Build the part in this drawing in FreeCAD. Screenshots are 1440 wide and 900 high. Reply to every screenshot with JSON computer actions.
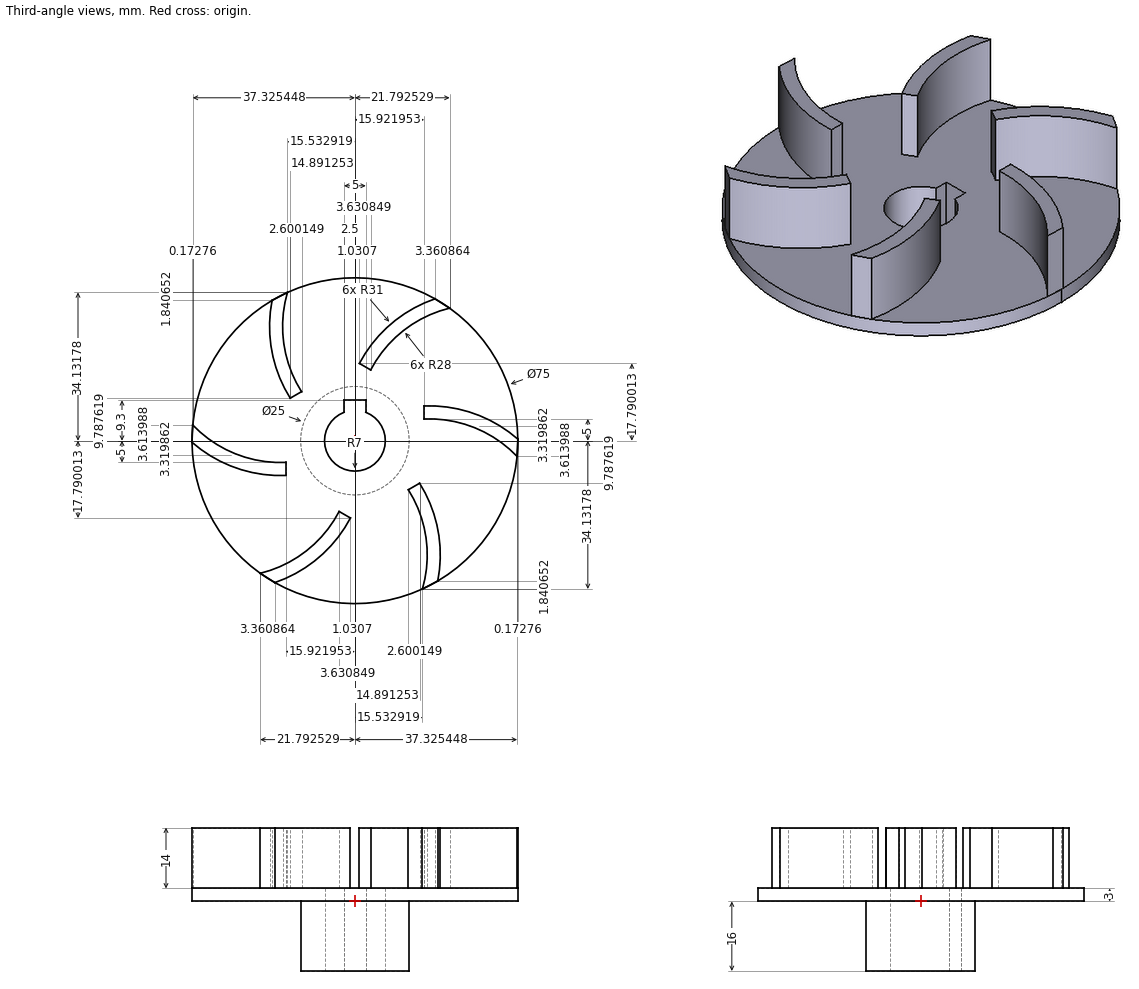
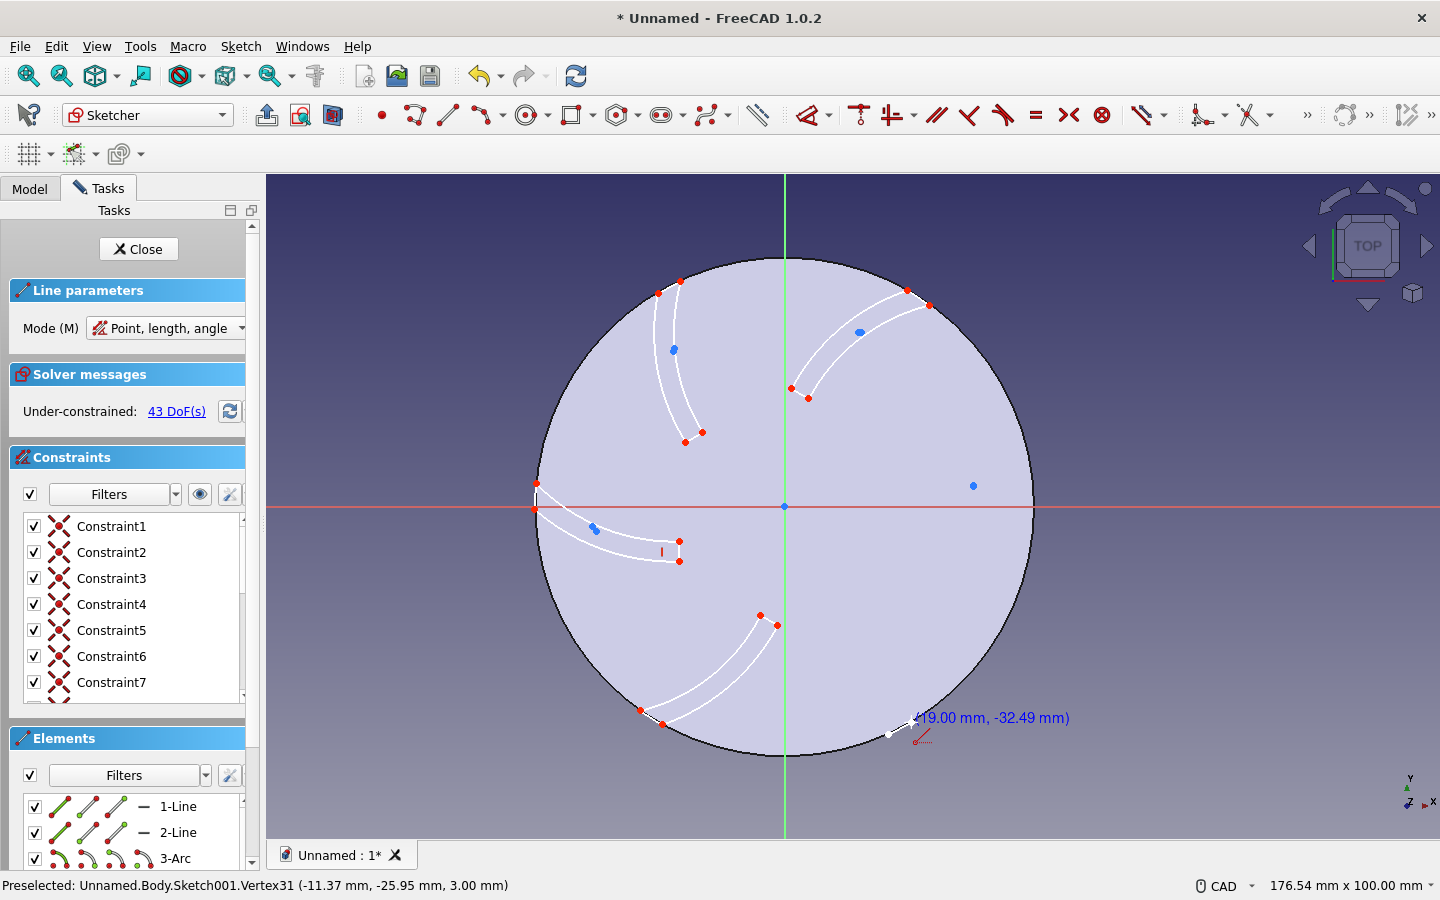
{"action": "left_click", "coordinate": [884, 572]}
{"action": "left_click", "coordinate": [866, 582]}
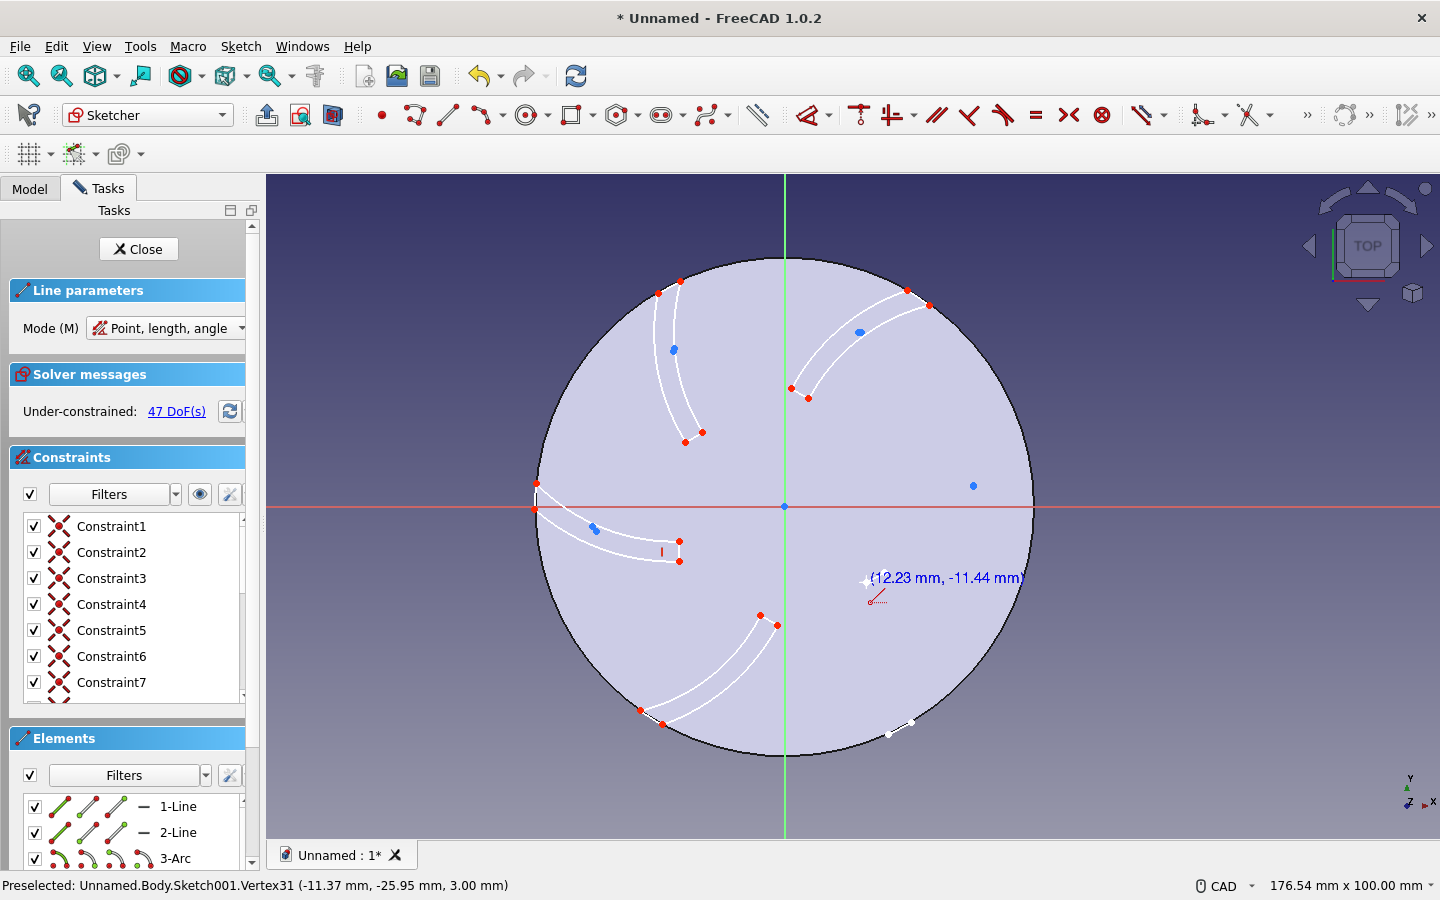
{"action": "left_click", "coordinate": [480, 116]}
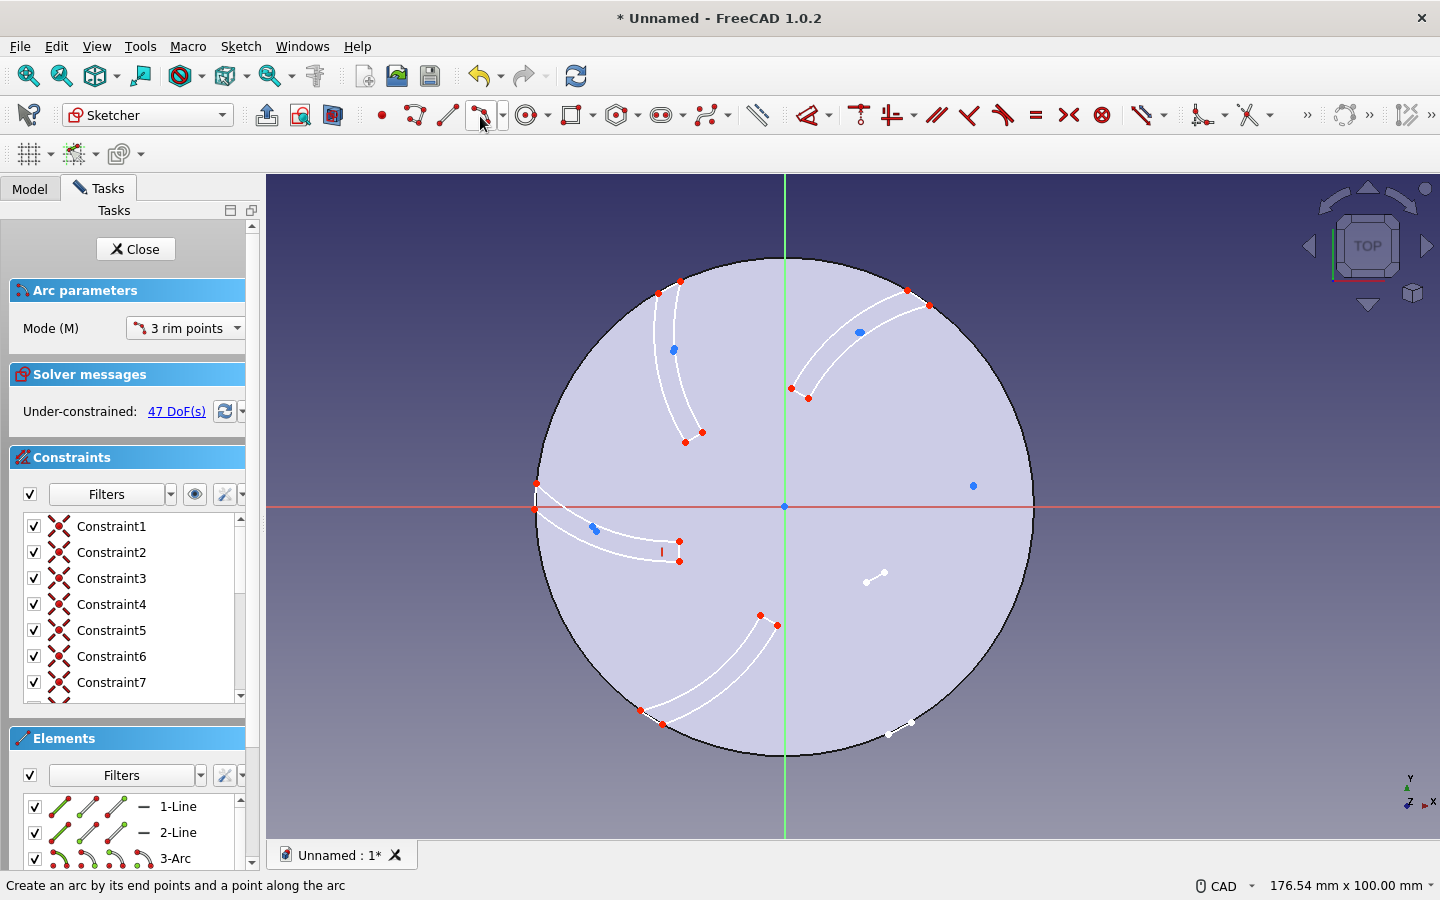
{"action": "left_click", "coordinate": [911, 723]}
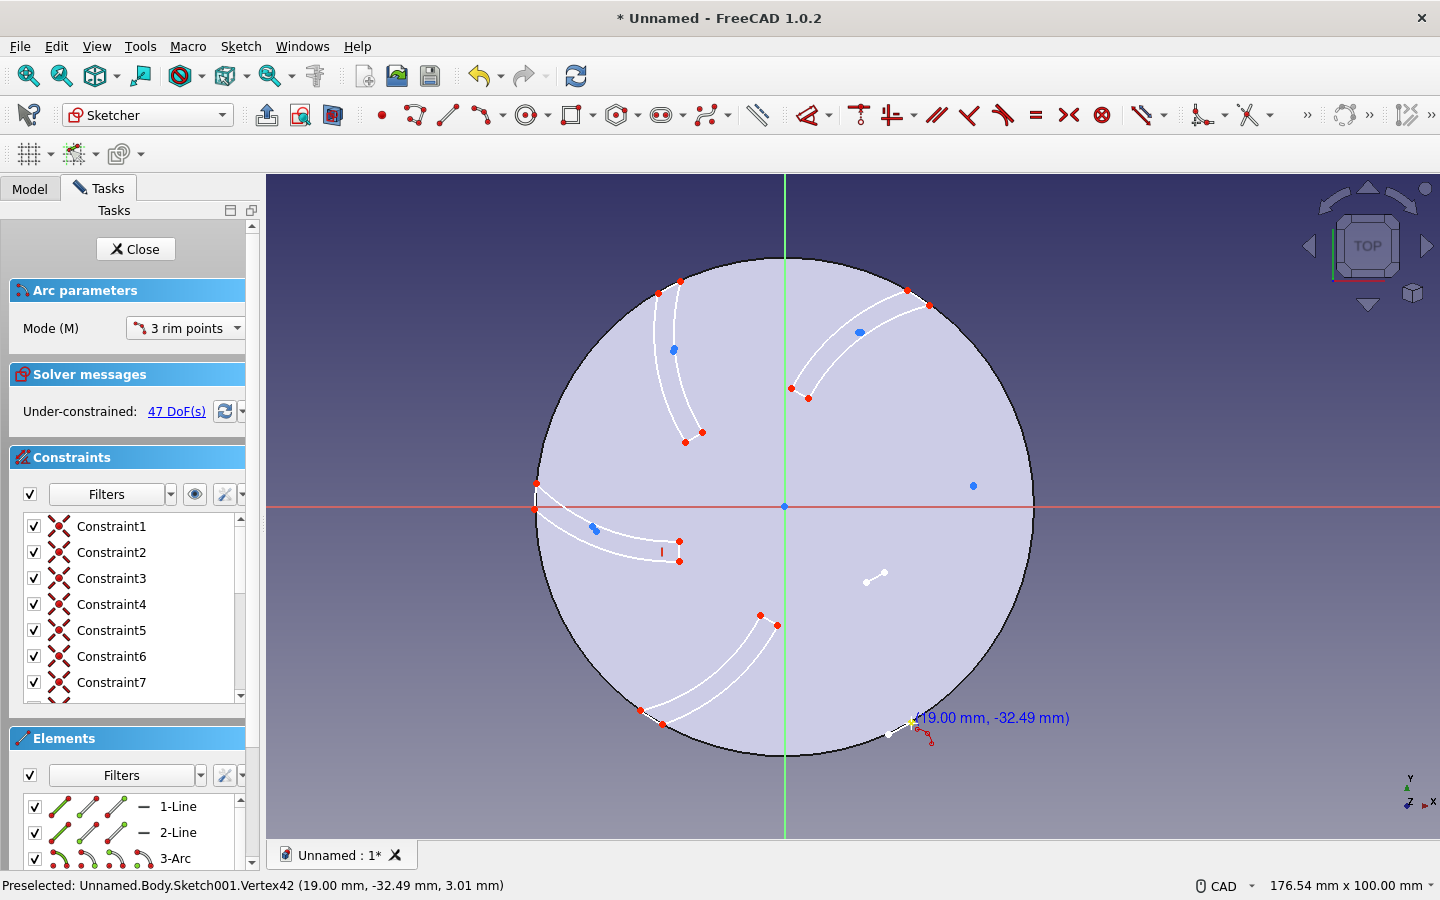
{"action": "scroll", "coordinate": [884, 572], "scroll_direction": "up", "scroll_amount": 3}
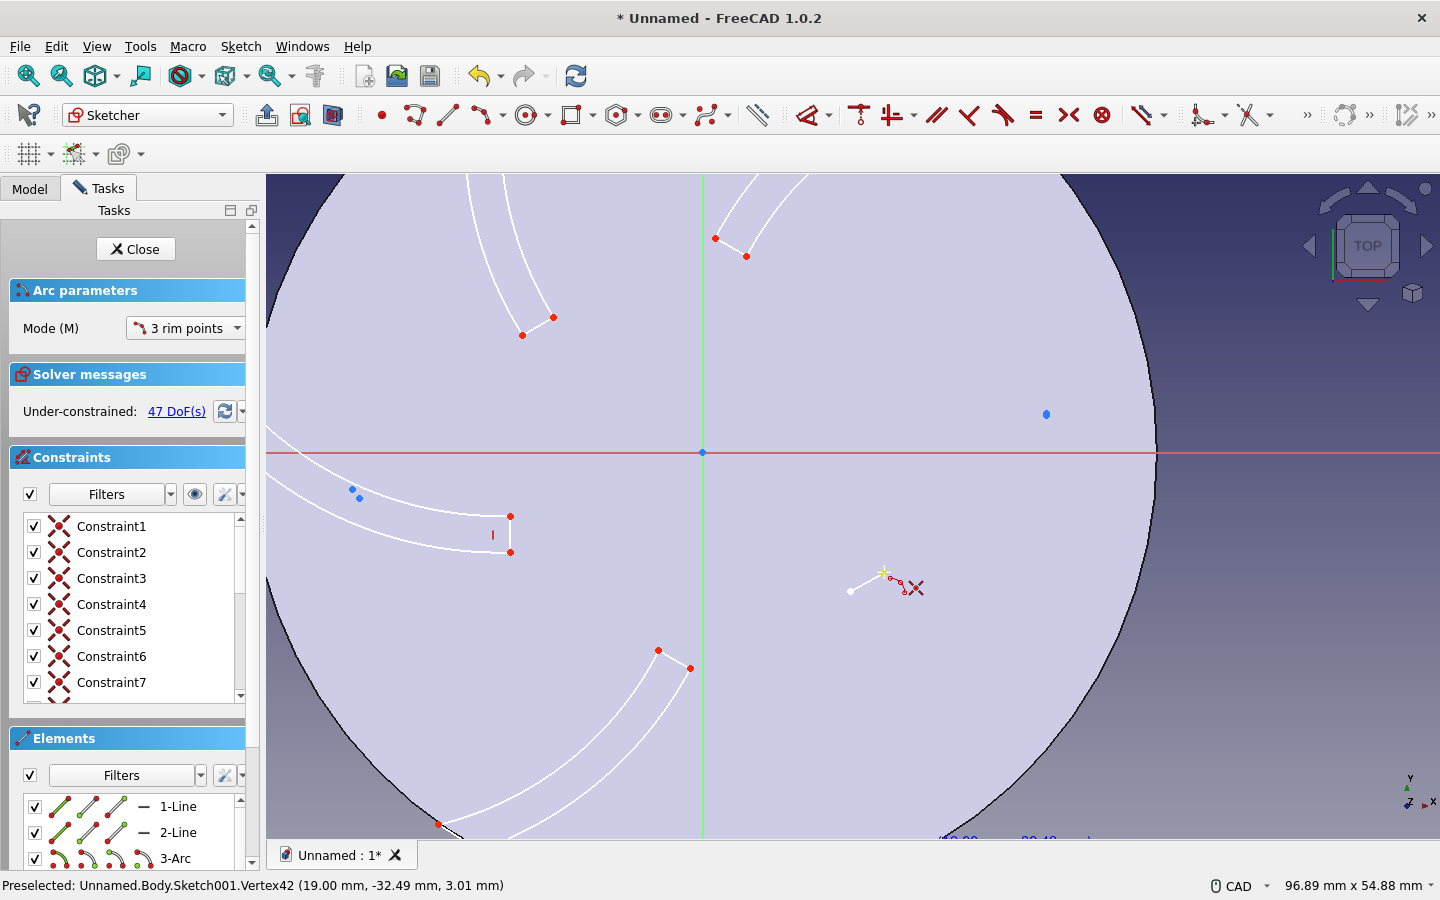
{"action": "left_click", "coordinate": [884, 573]}
{"action": "left_click", "coordinate": [934, 703]}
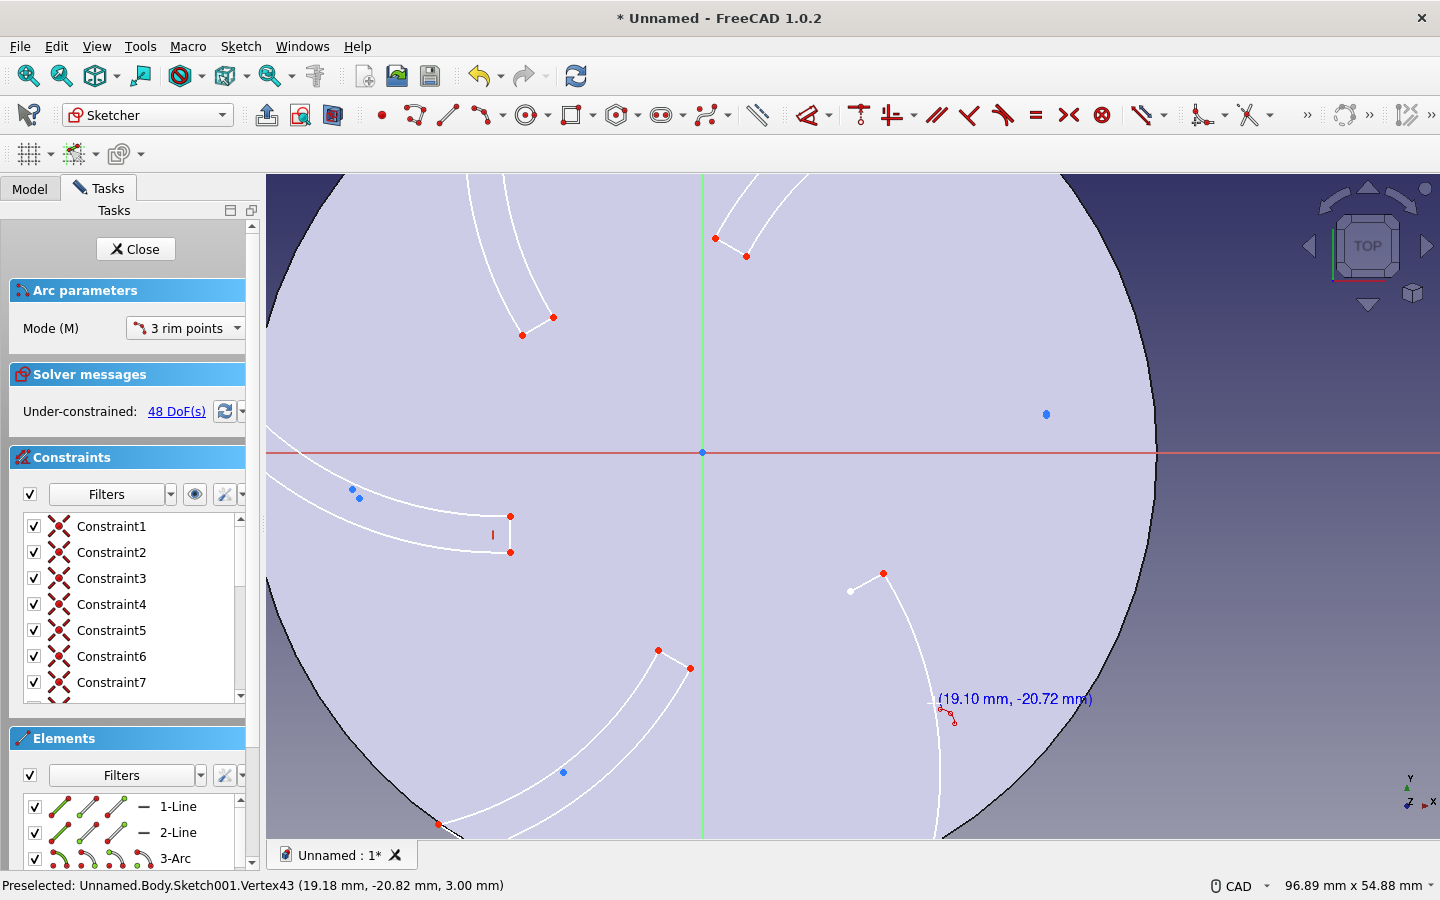
{"action": "left_click", "coordinate": [851, 592]}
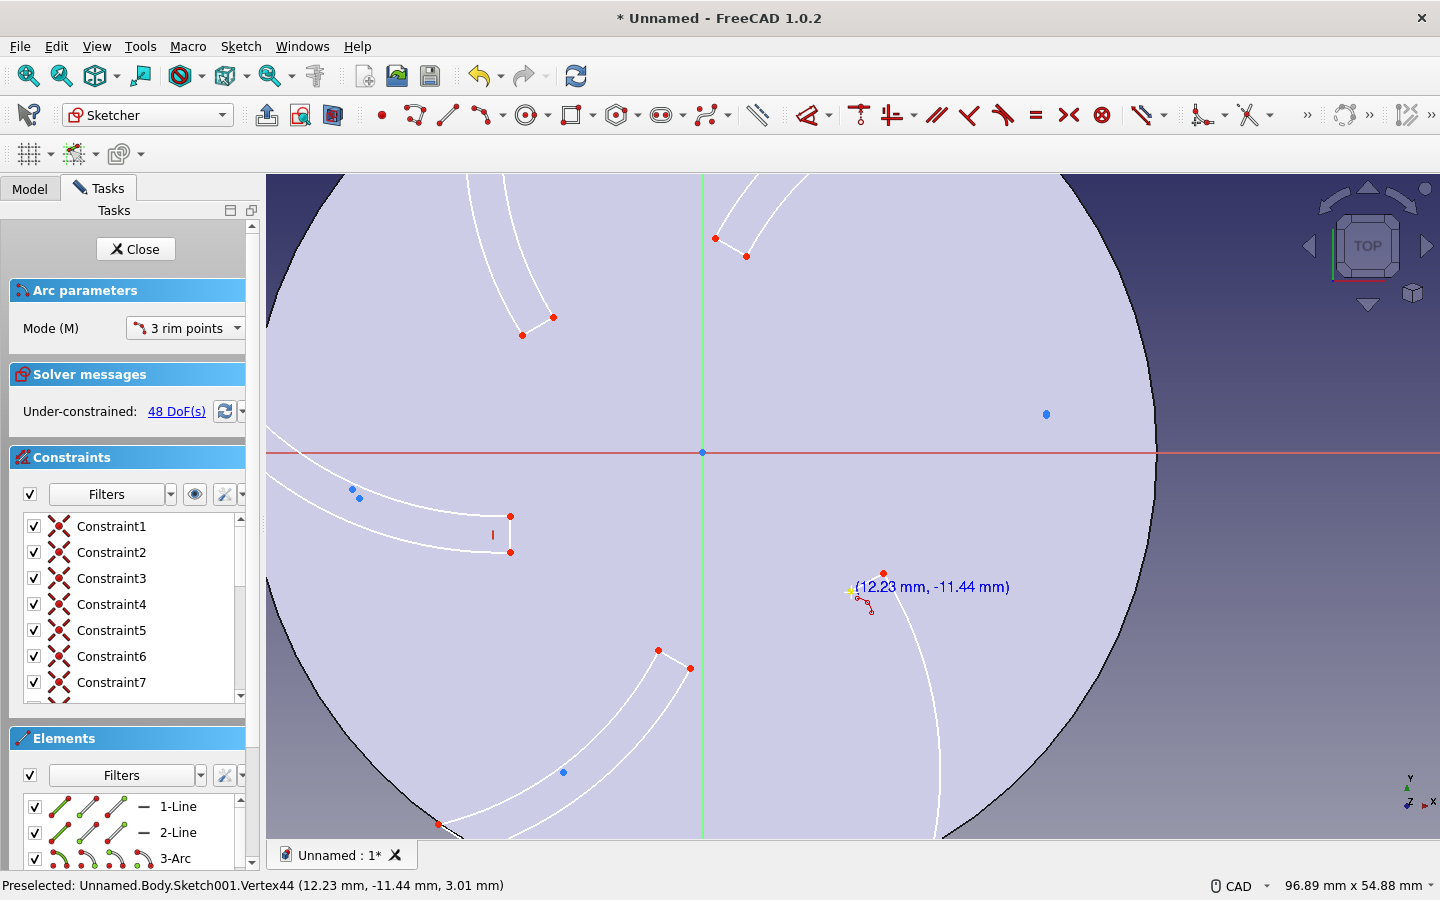
{"action": "scroll", "coordinate": [884, 572], "scroll_direction": "down", "scroll_amount": 3}